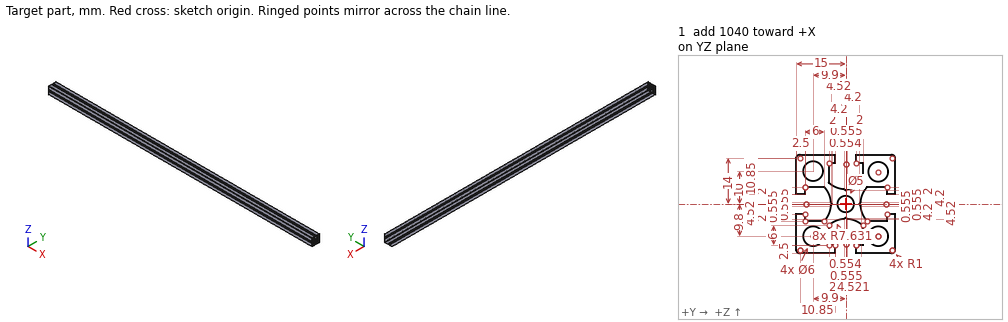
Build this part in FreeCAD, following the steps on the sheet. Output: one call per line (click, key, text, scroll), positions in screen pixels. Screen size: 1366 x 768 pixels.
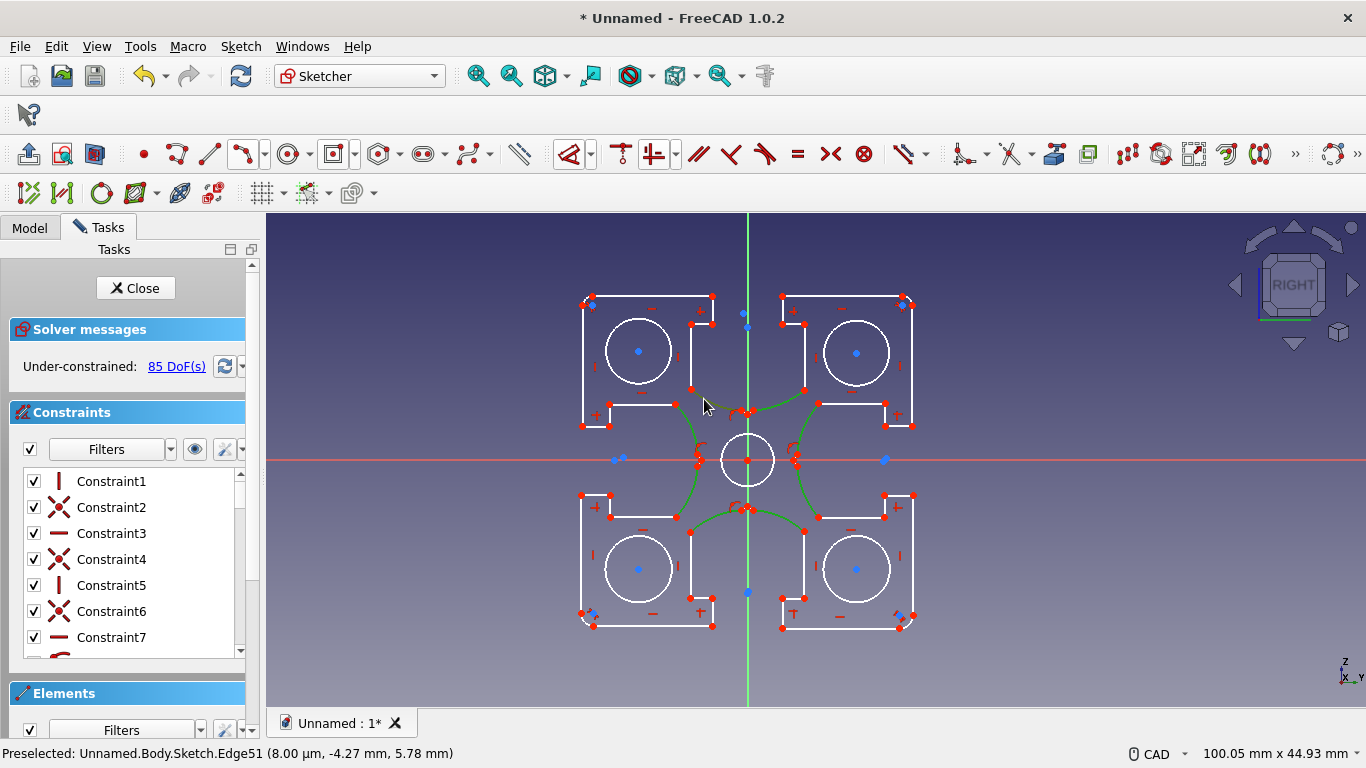
click(798, 154)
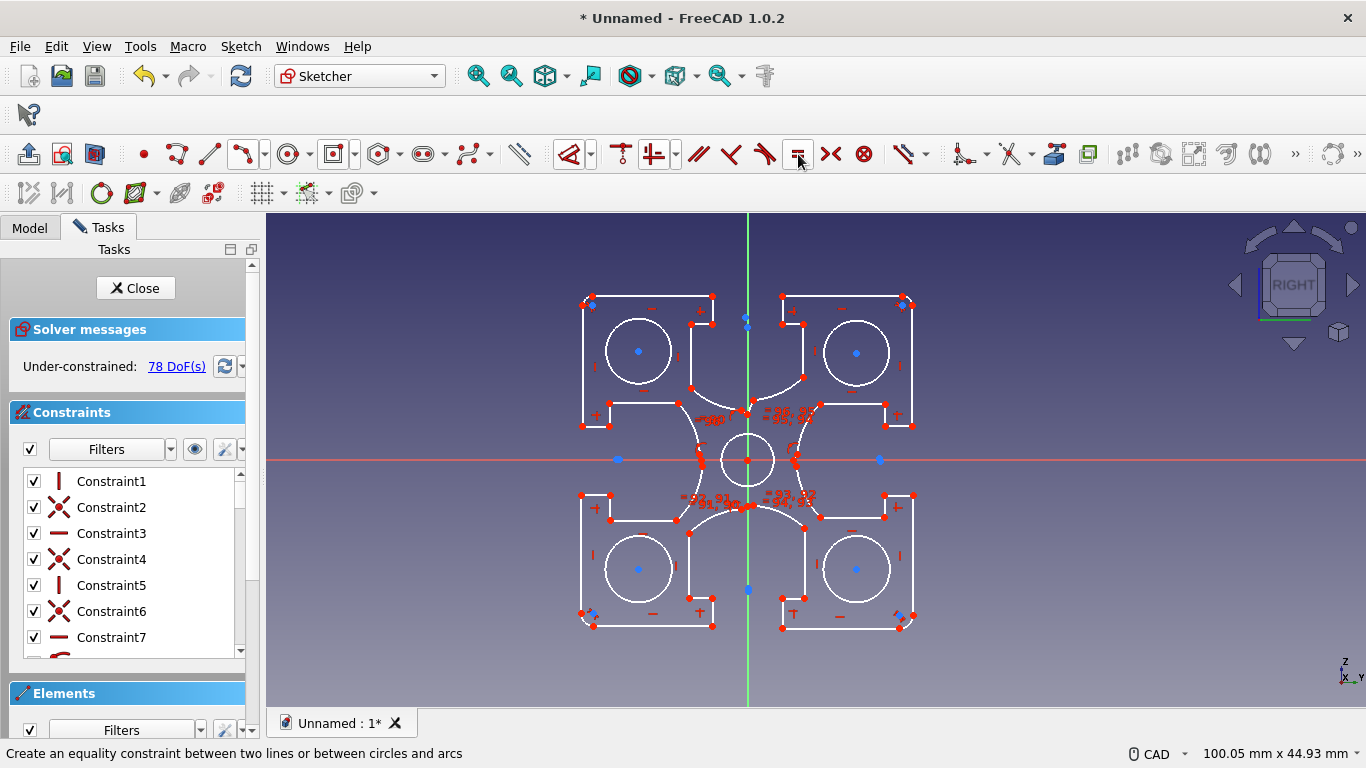
scroll(585, 622, up, 2)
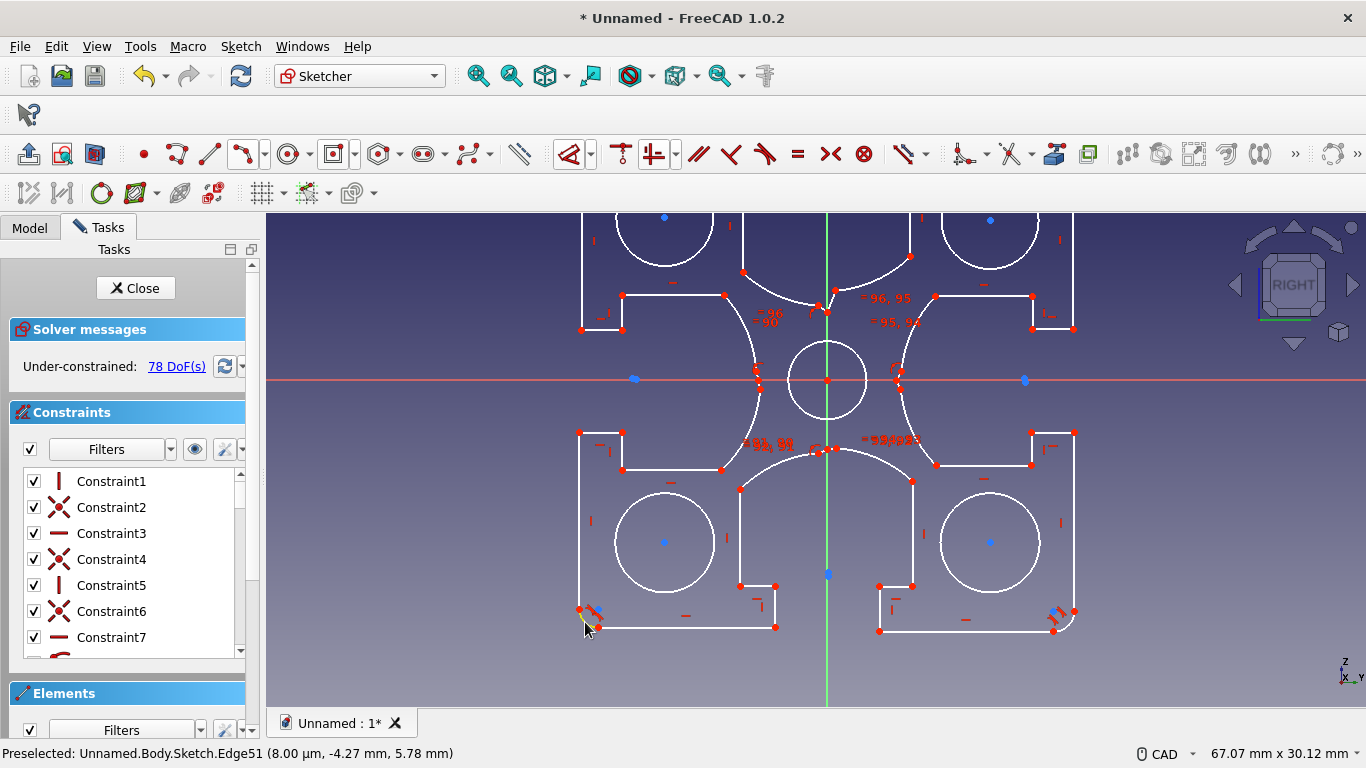
click(585, 622)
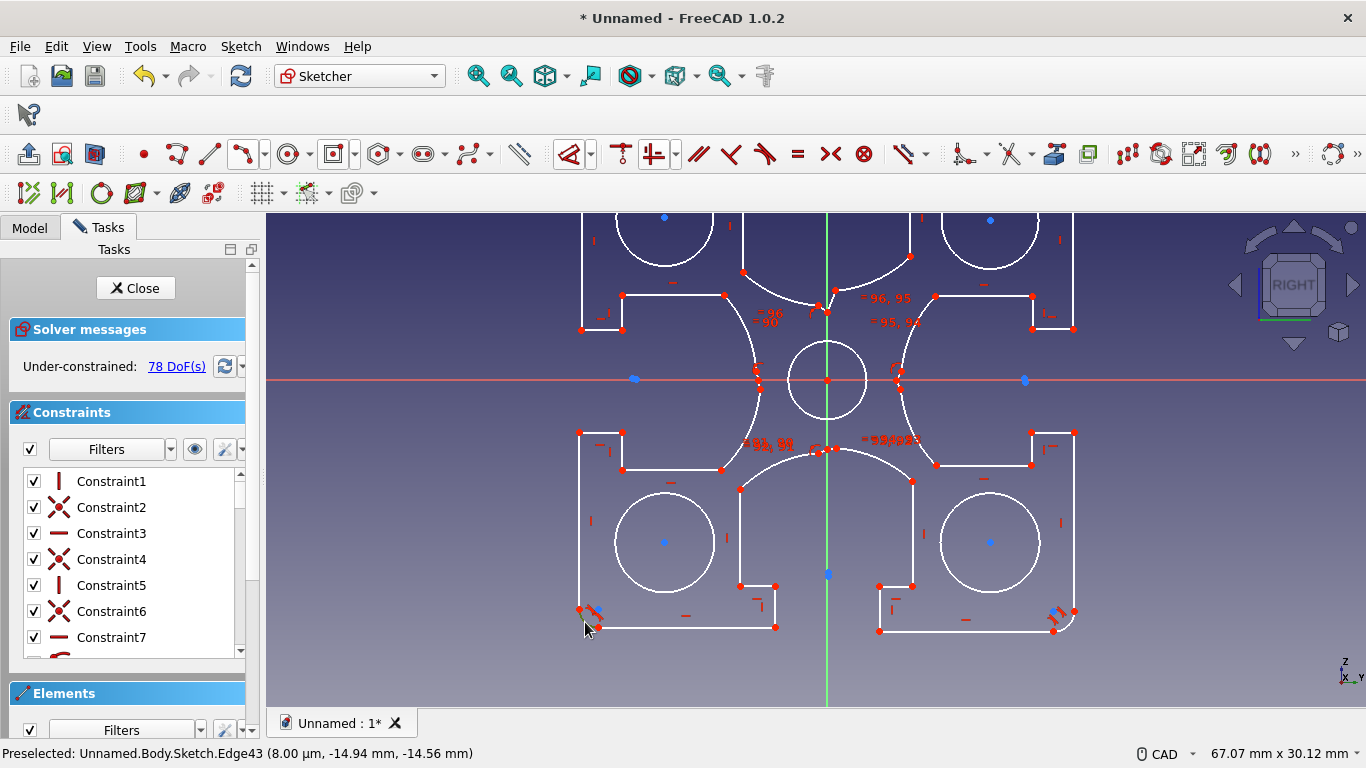
scroll(1063, 629, up, 2)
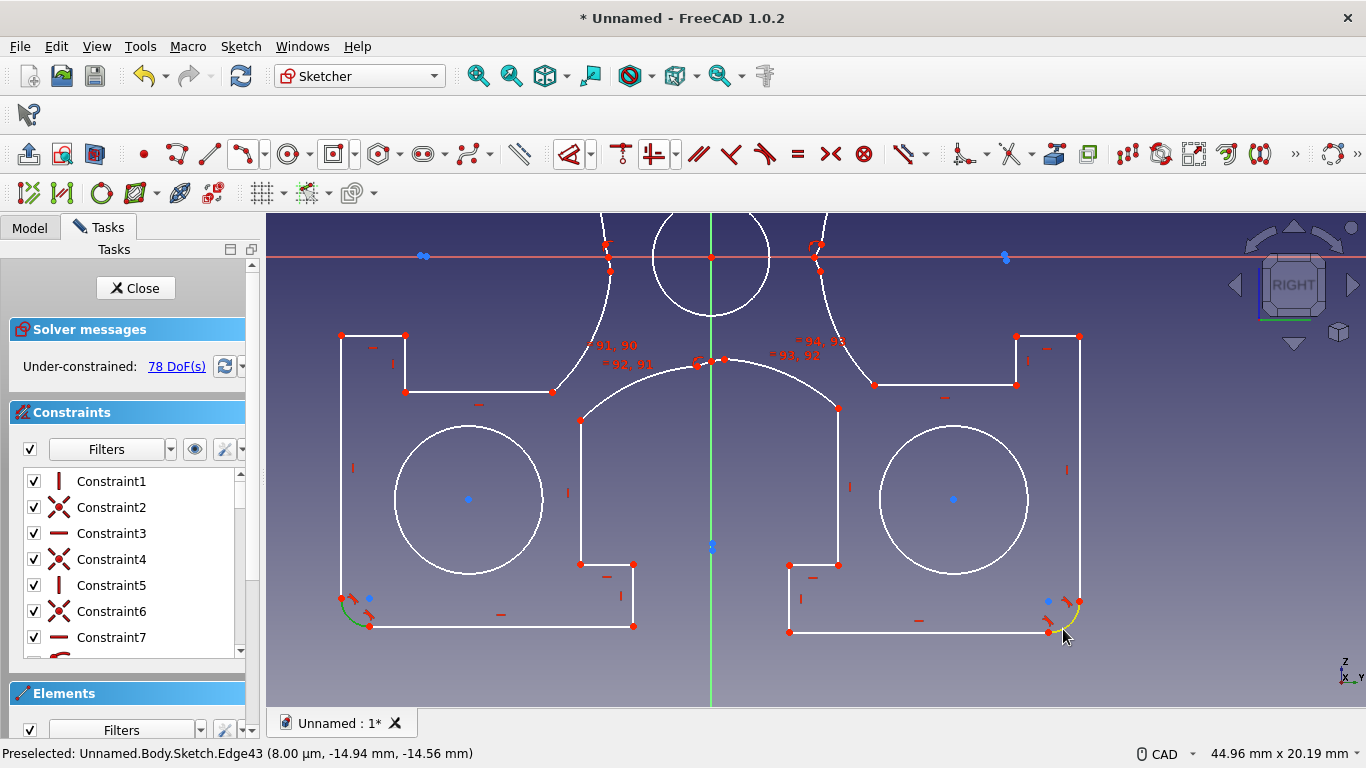
click(1063, 629)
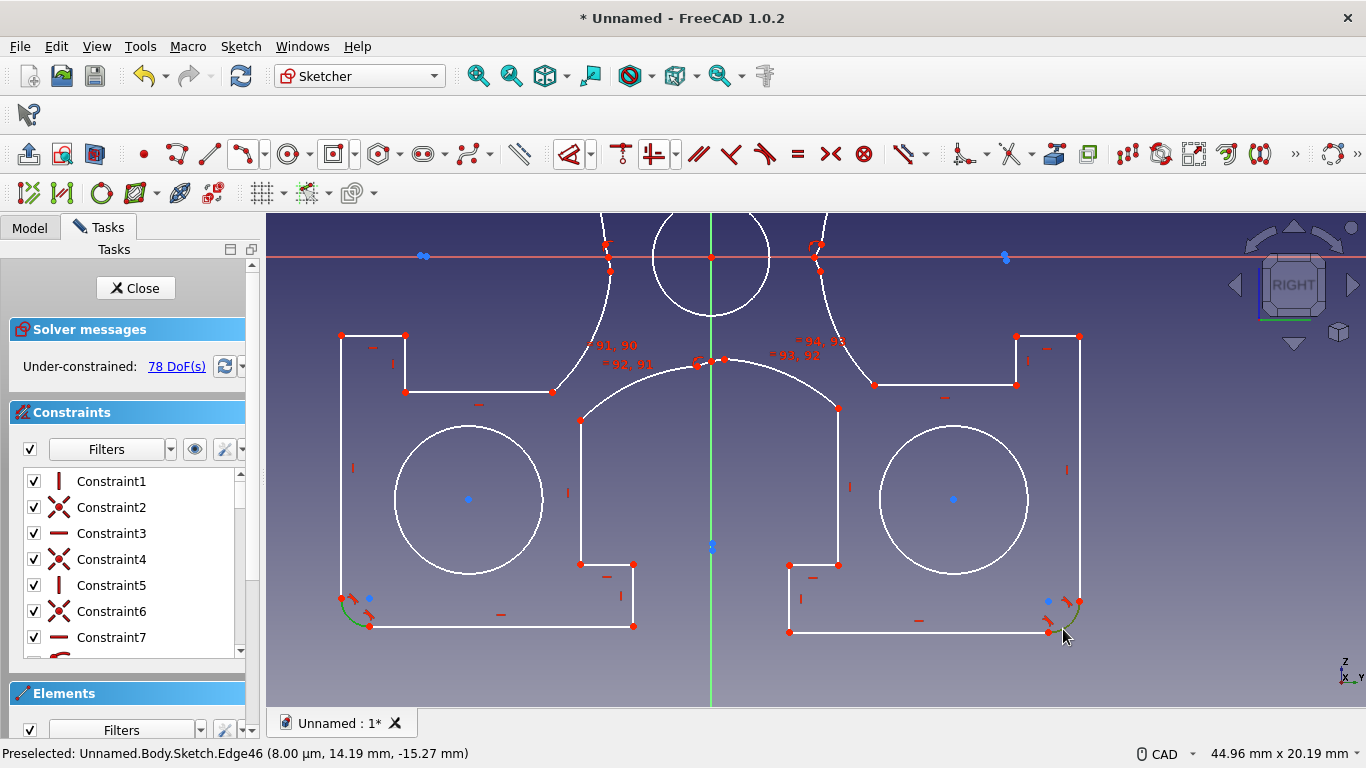
scroll(777, 625, down, 4)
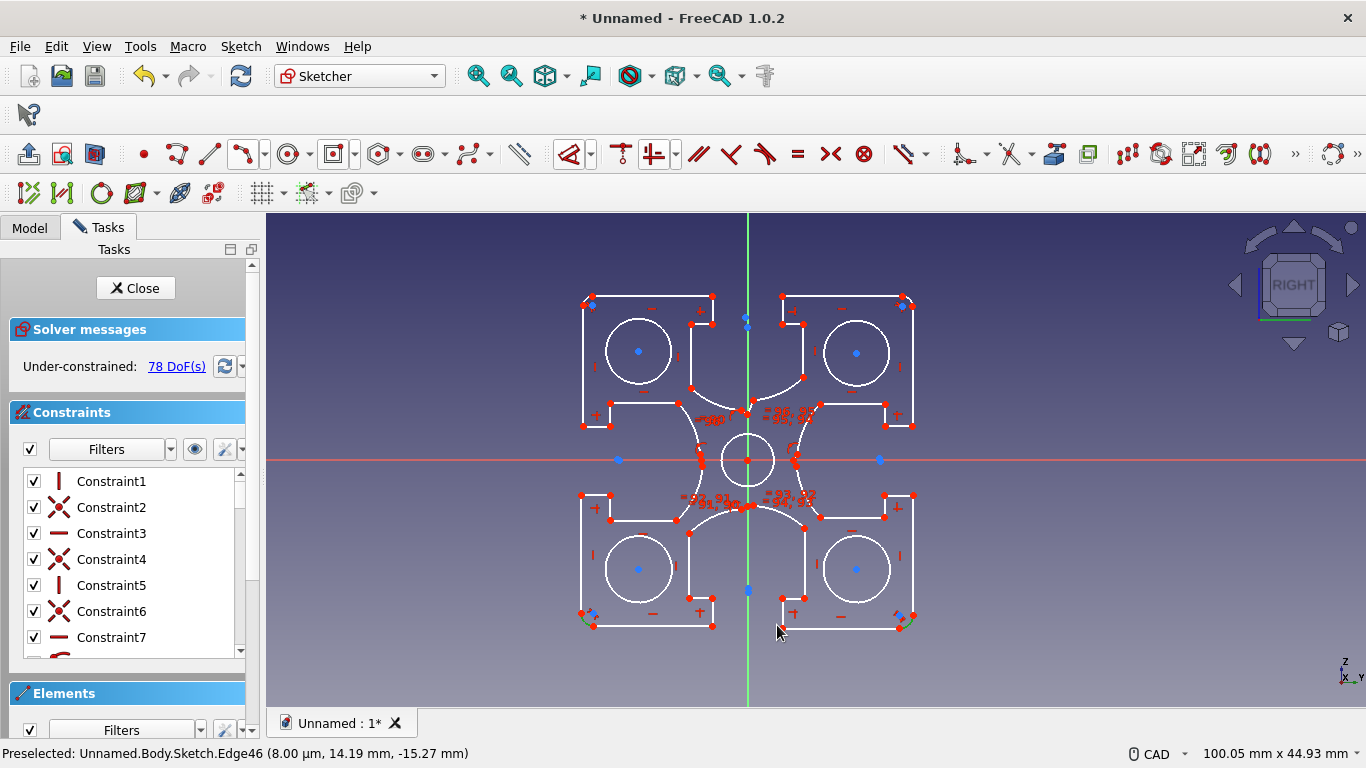
scroll(911, 302, up, 6)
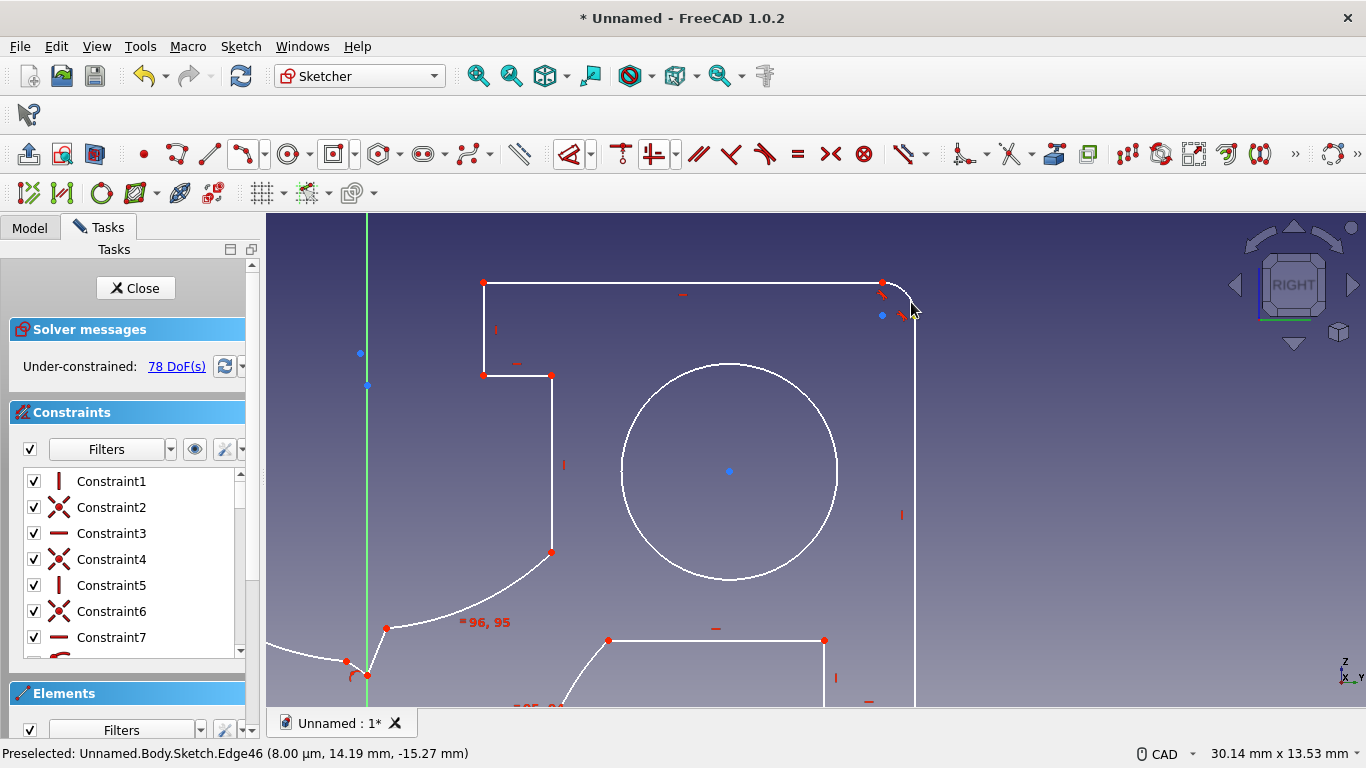
click(911, 300)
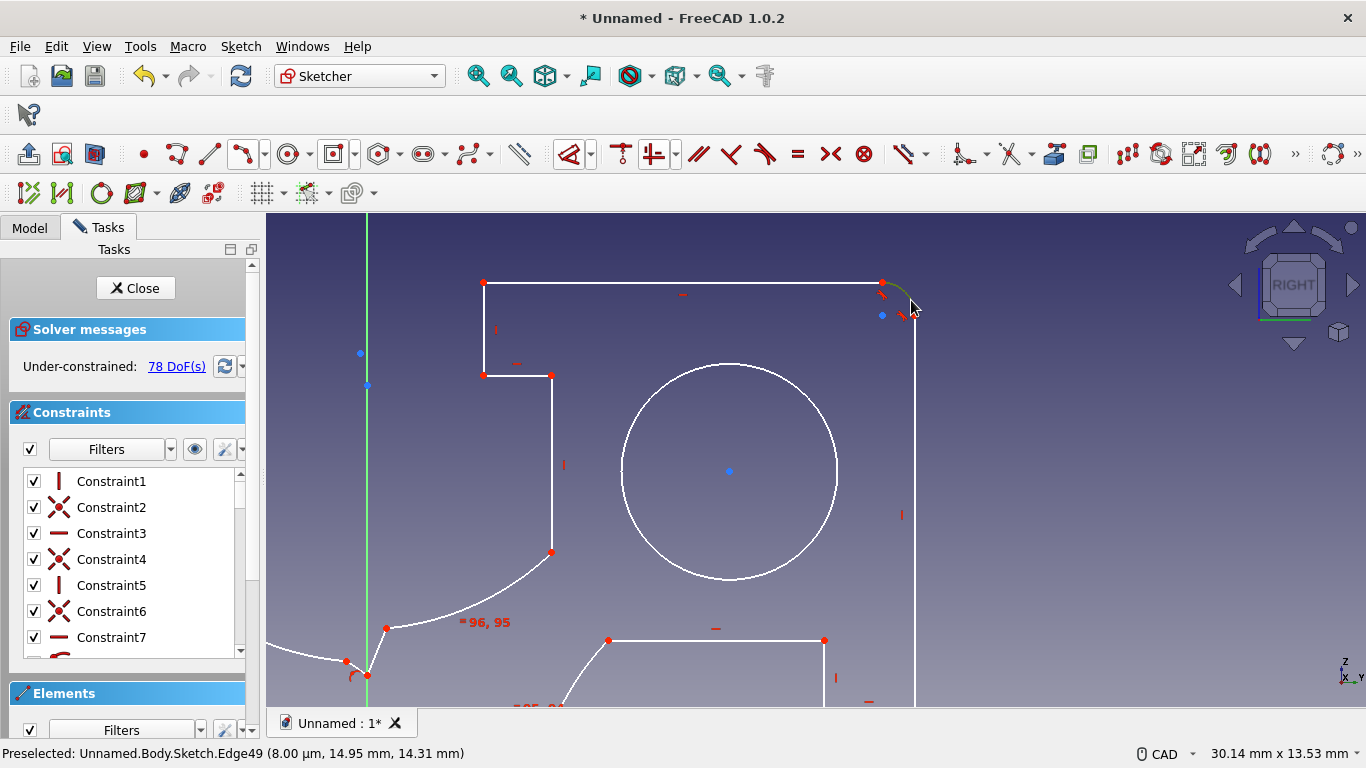
scroll(911, 302, down, 6)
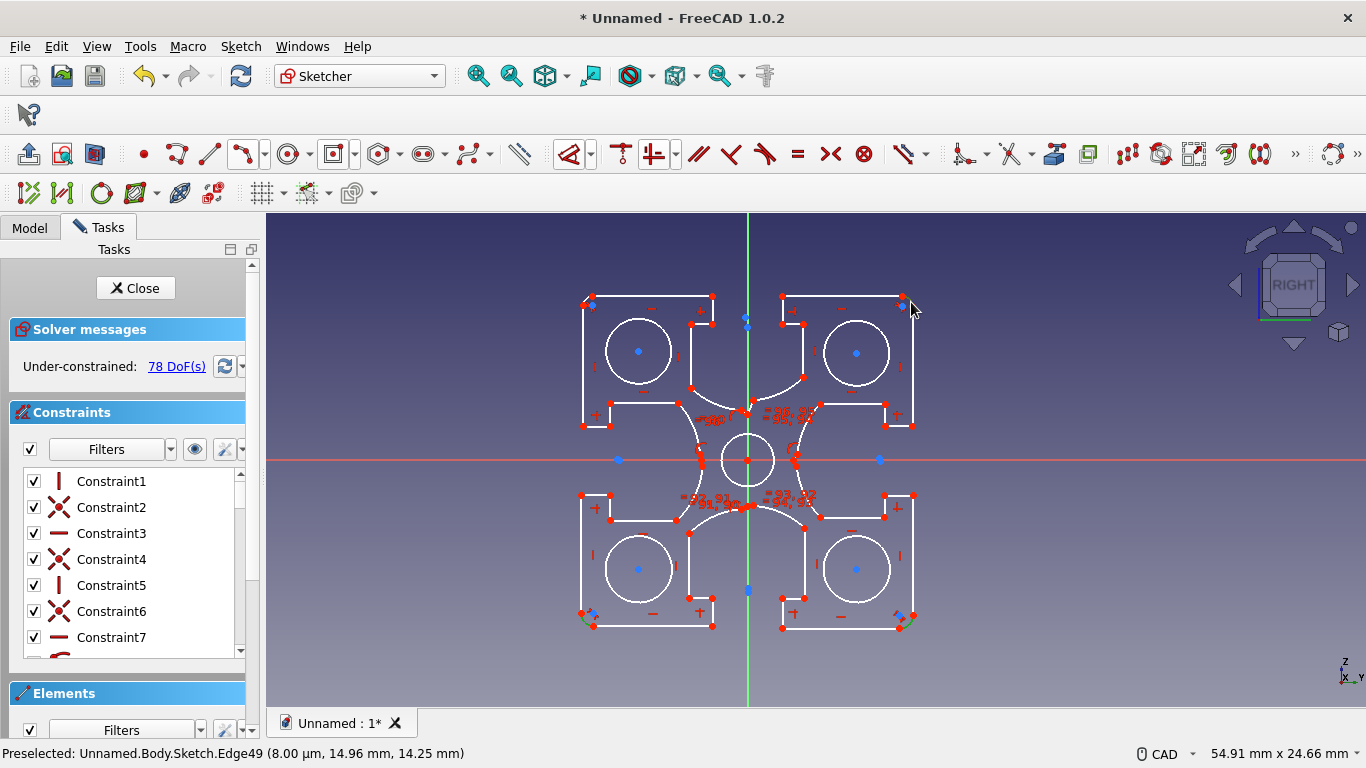
scroll(588, 297, up, 6)